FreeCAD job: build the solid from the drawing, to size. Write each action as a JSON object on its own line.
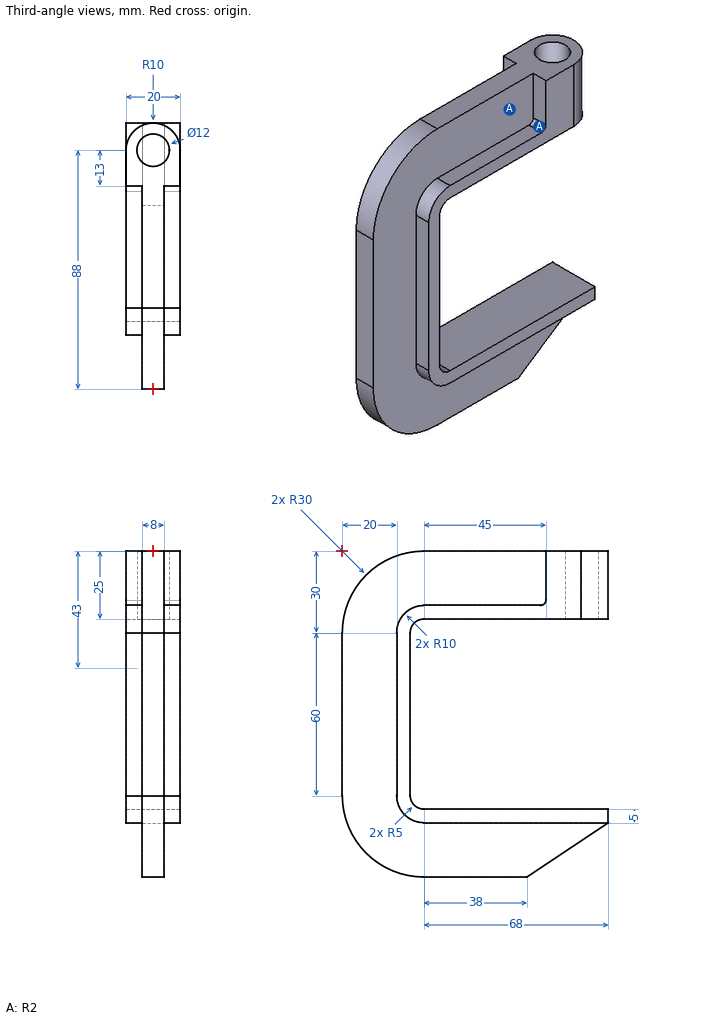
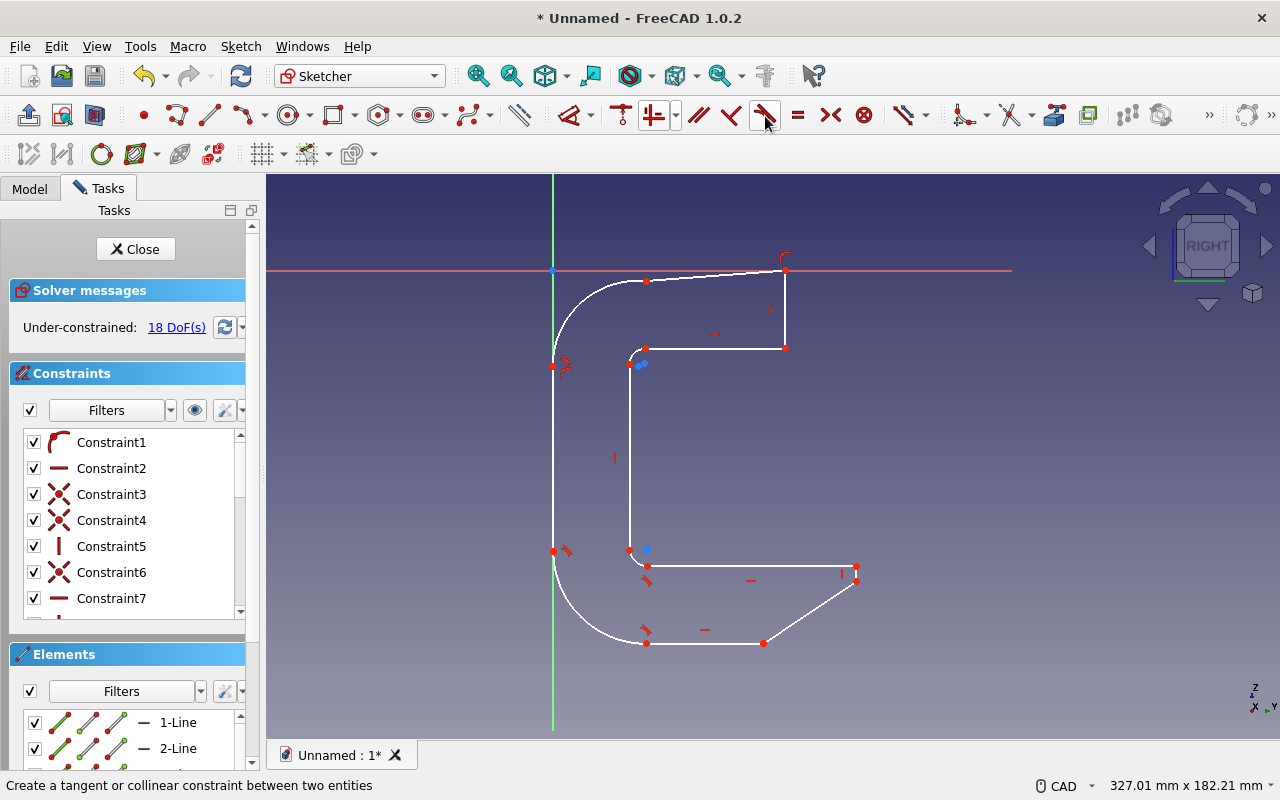
{"action": "left_click", "coordinate": [630, 495]}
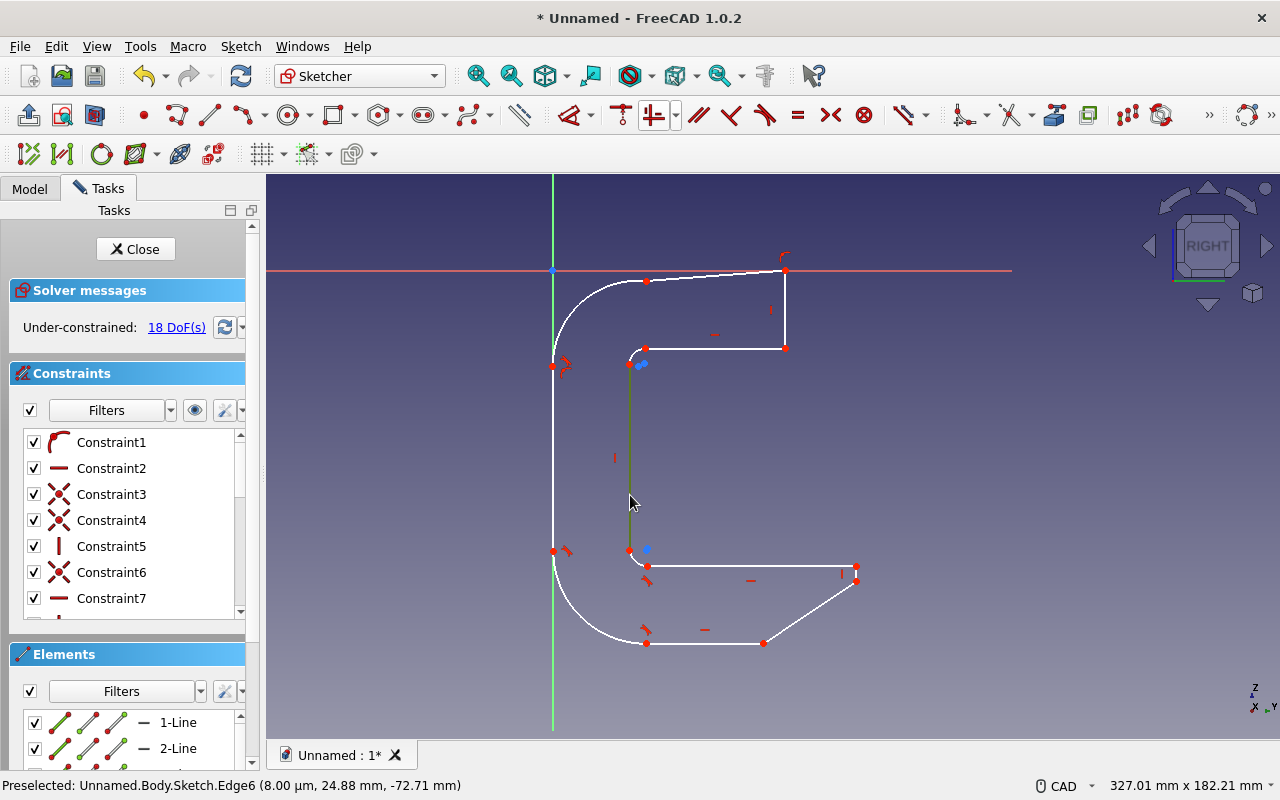
{"action": "left_click", "coordinate": [636, 562]}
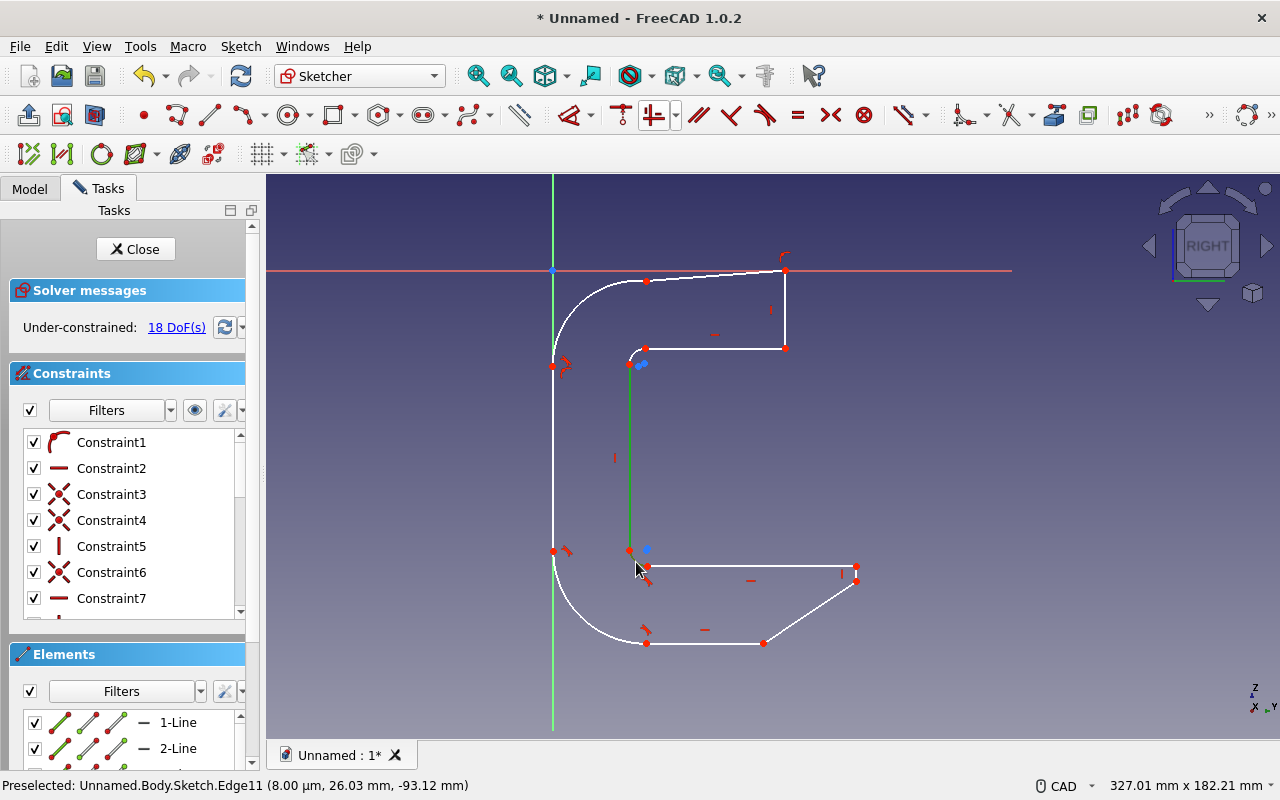
{"action": "key", "text": "t"}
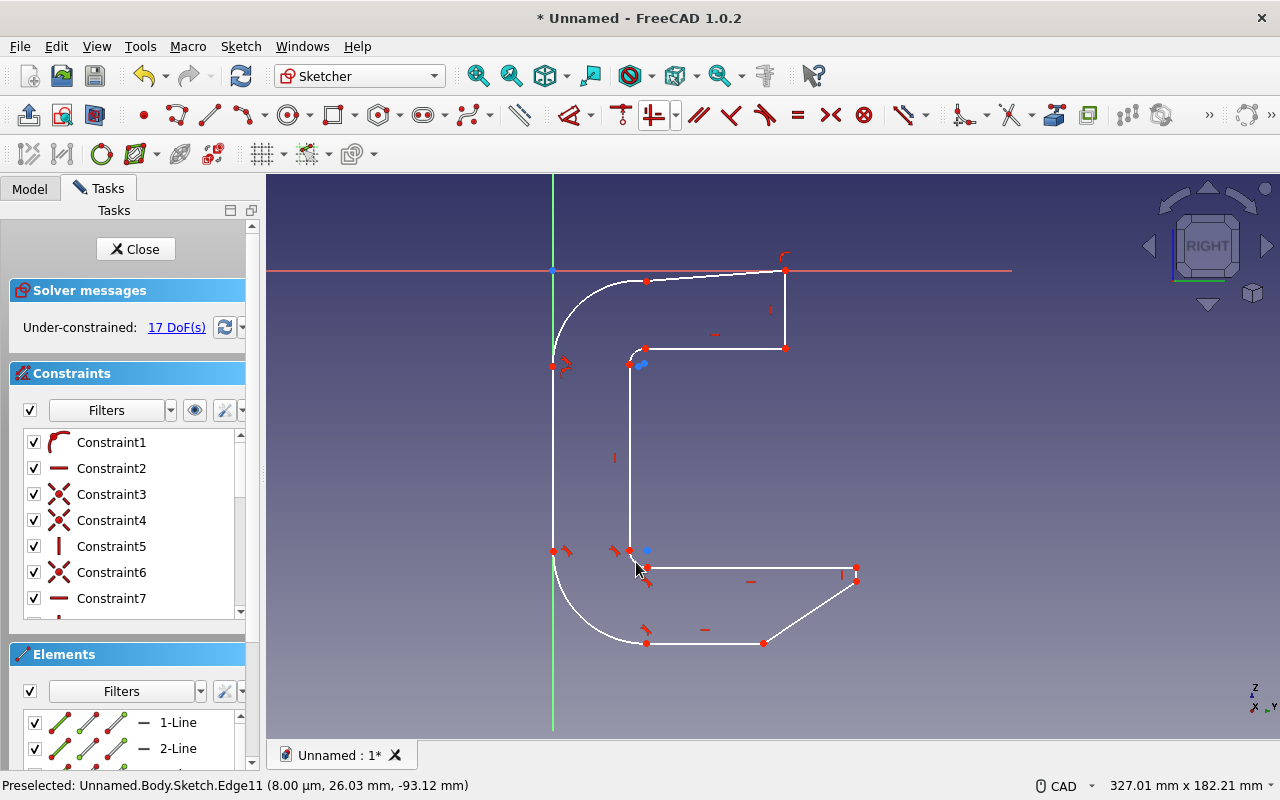
{"action": "left_click", "coordinate": [630, 495]}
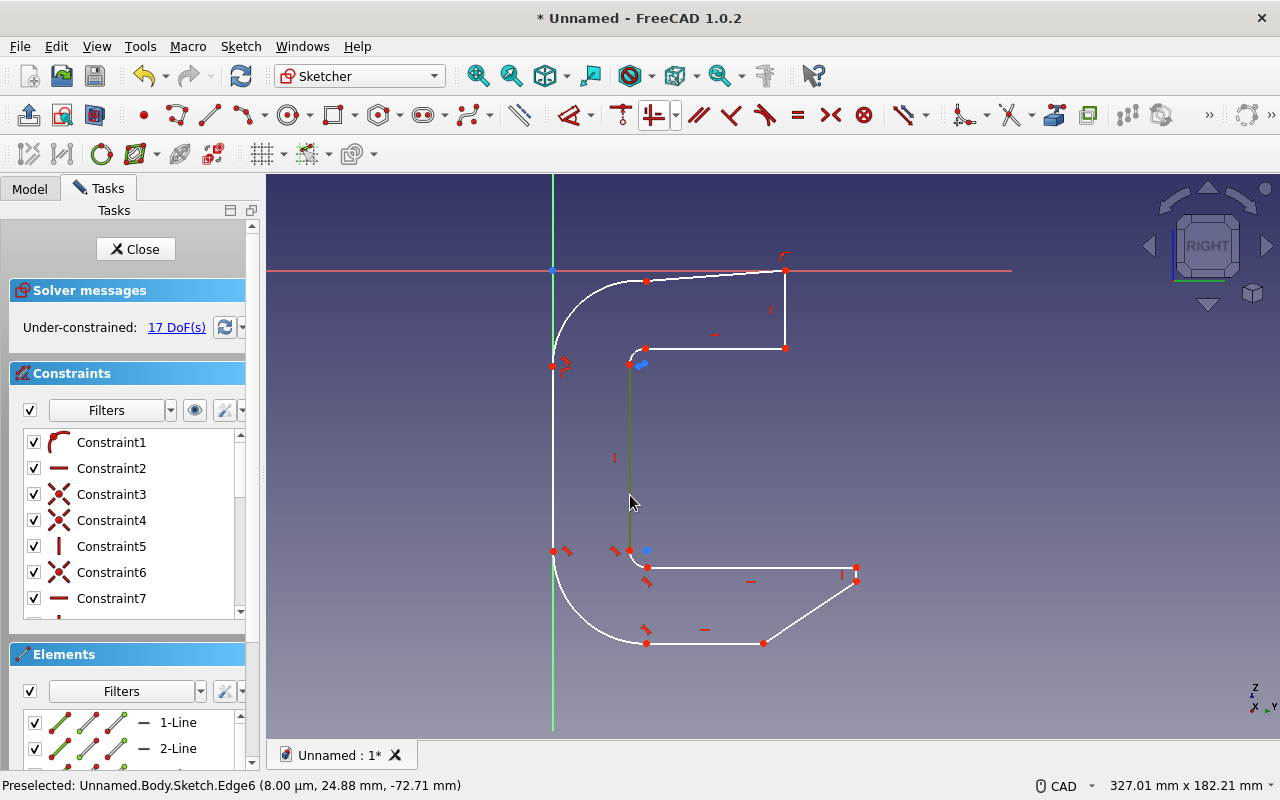
{"action": "left_click", "coordinate": [634, 353]}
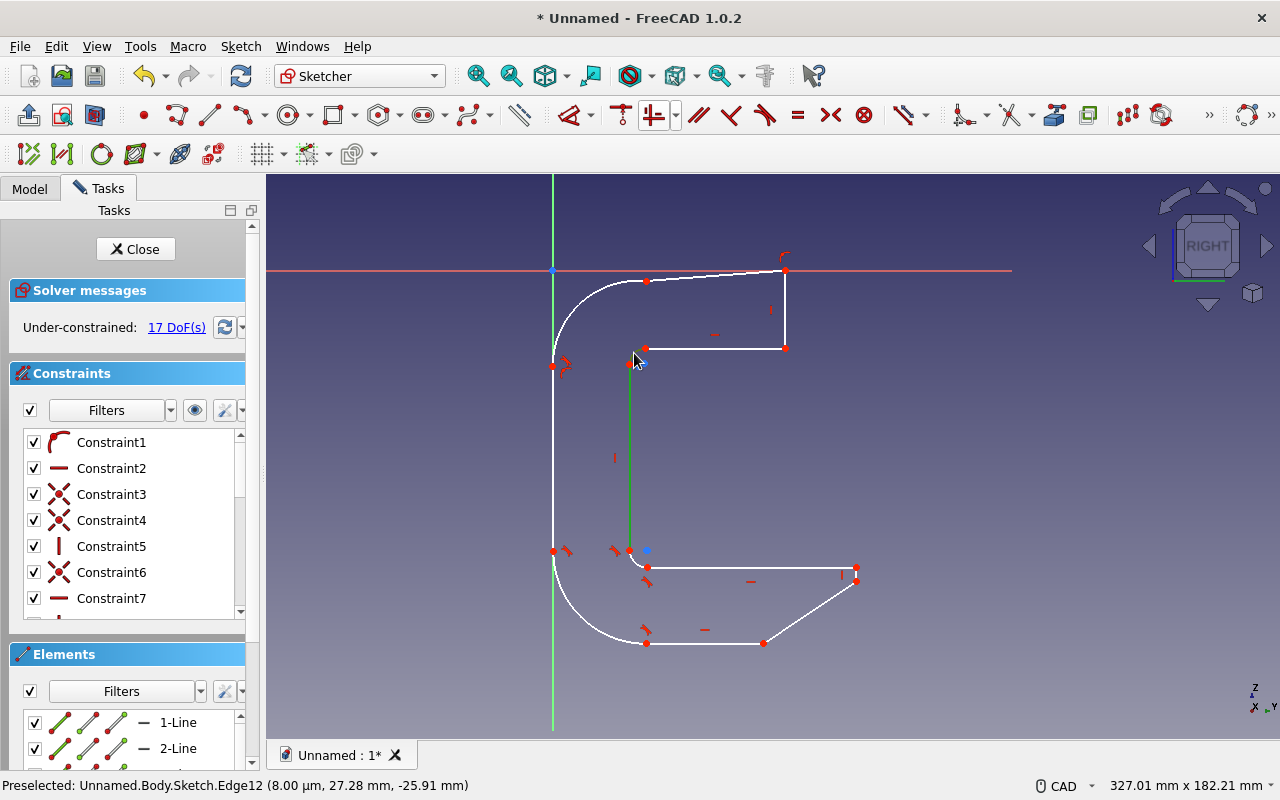
{"action": "left_click", "coordinate": [765, 116]}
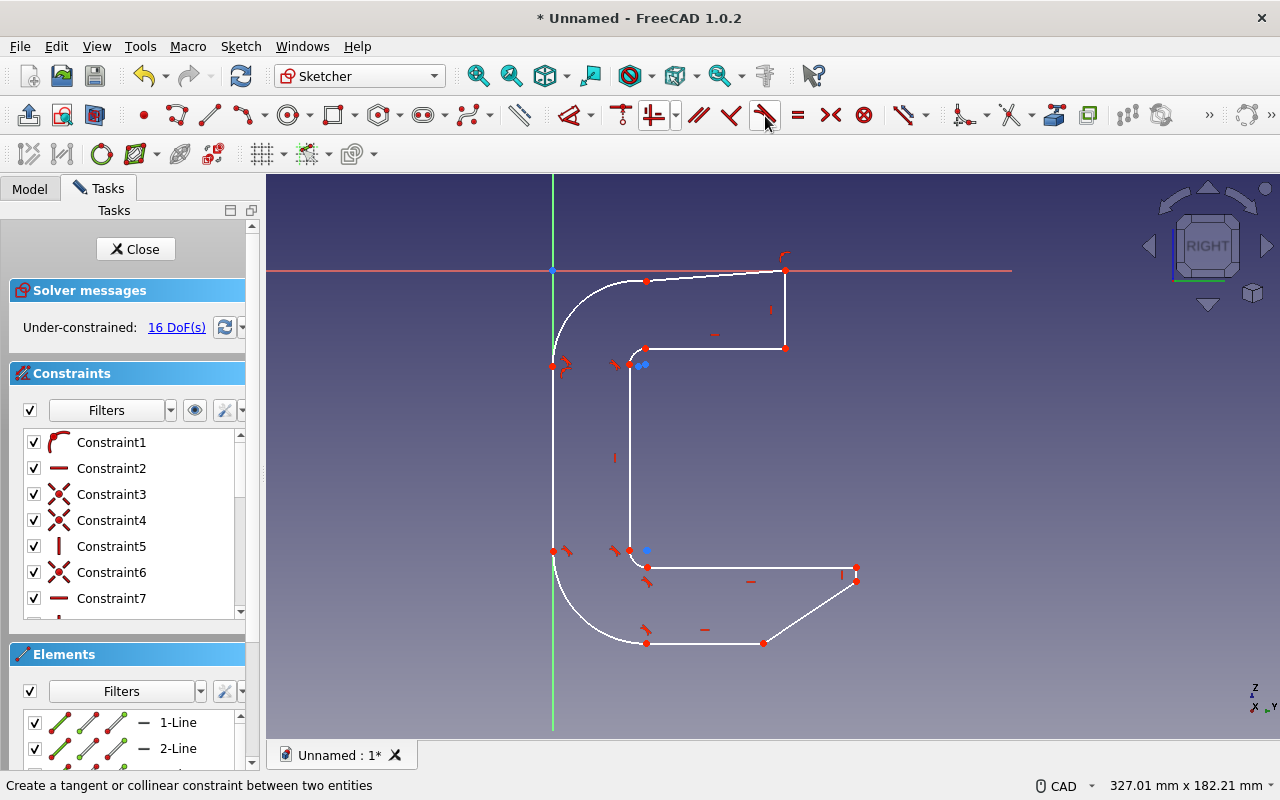
{"action": "left_click", "coordinate": [687, 349]}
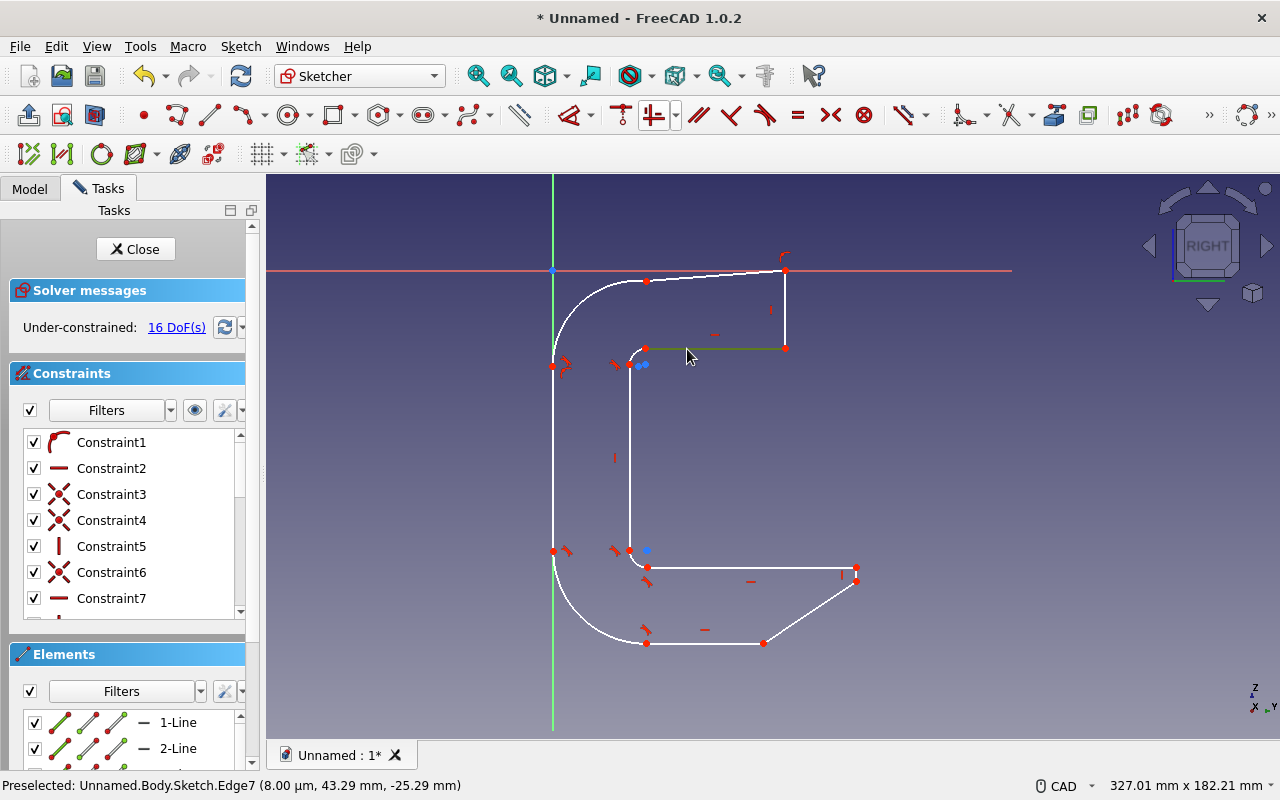
{"action": "left_click", "coordinate": [634, 354]}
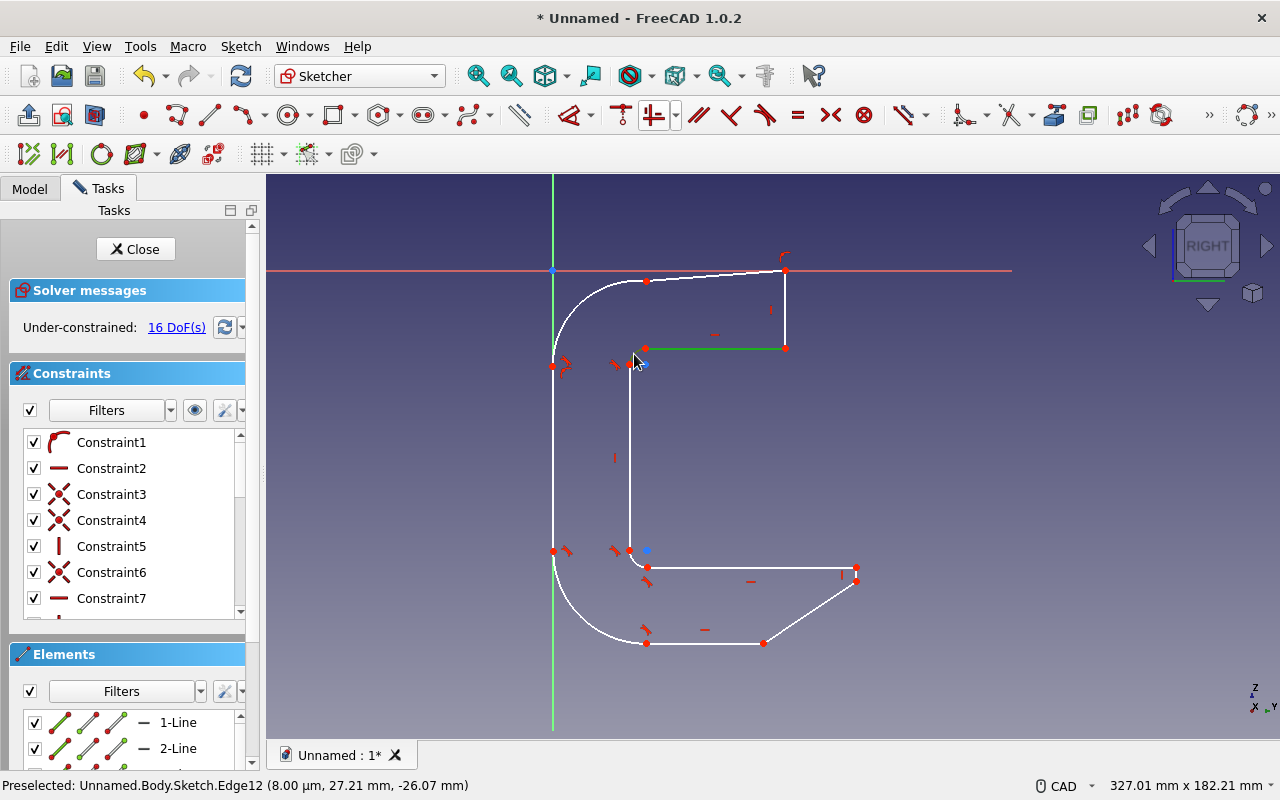
{"action": "left_click", "coordinate": [765, 116]}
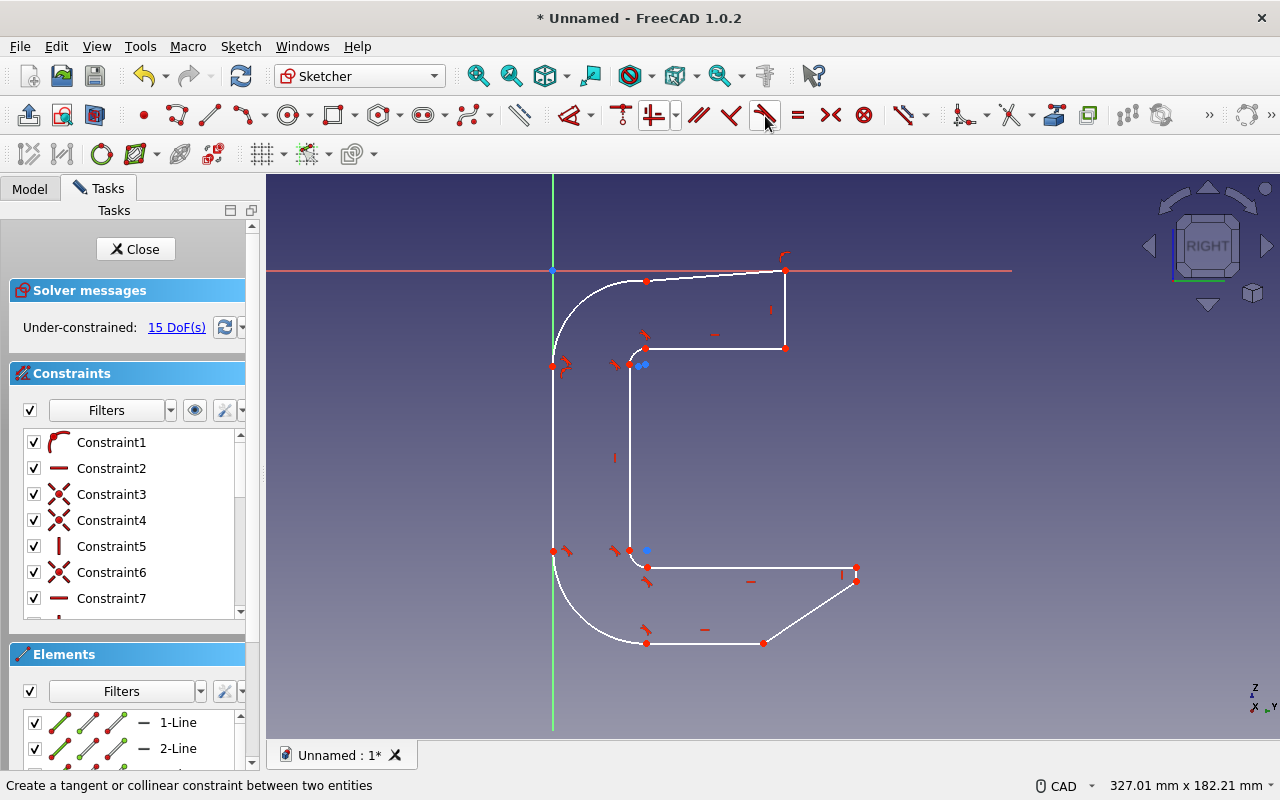
{"action": "left_click", "coordinate": [744, 274]}